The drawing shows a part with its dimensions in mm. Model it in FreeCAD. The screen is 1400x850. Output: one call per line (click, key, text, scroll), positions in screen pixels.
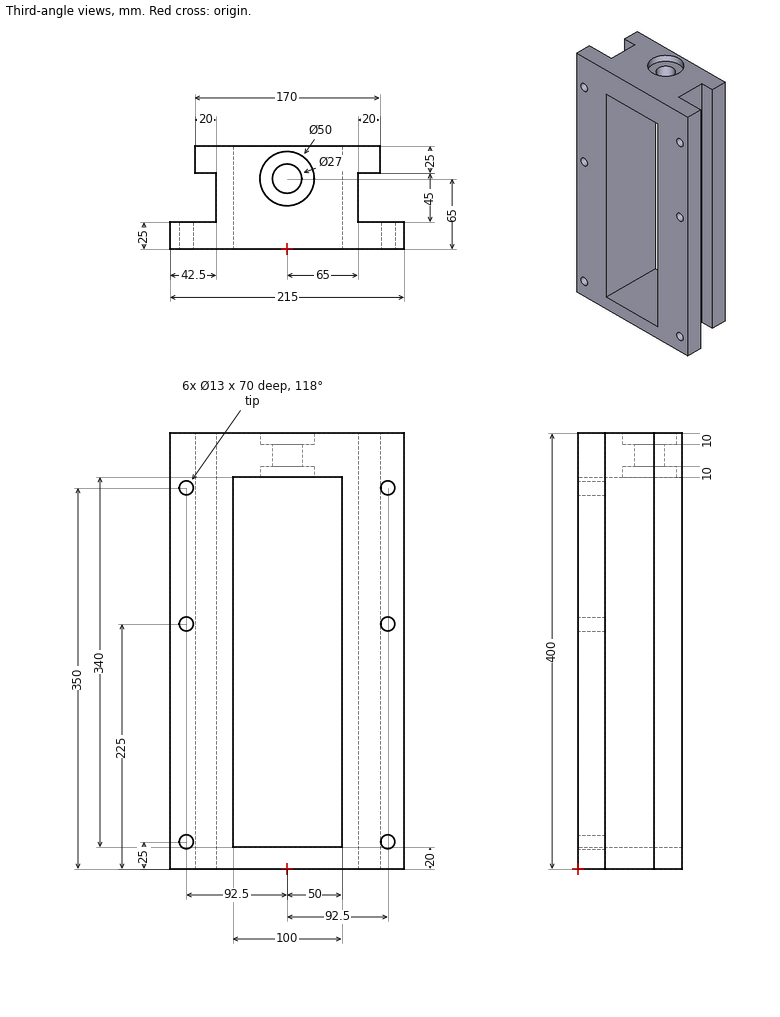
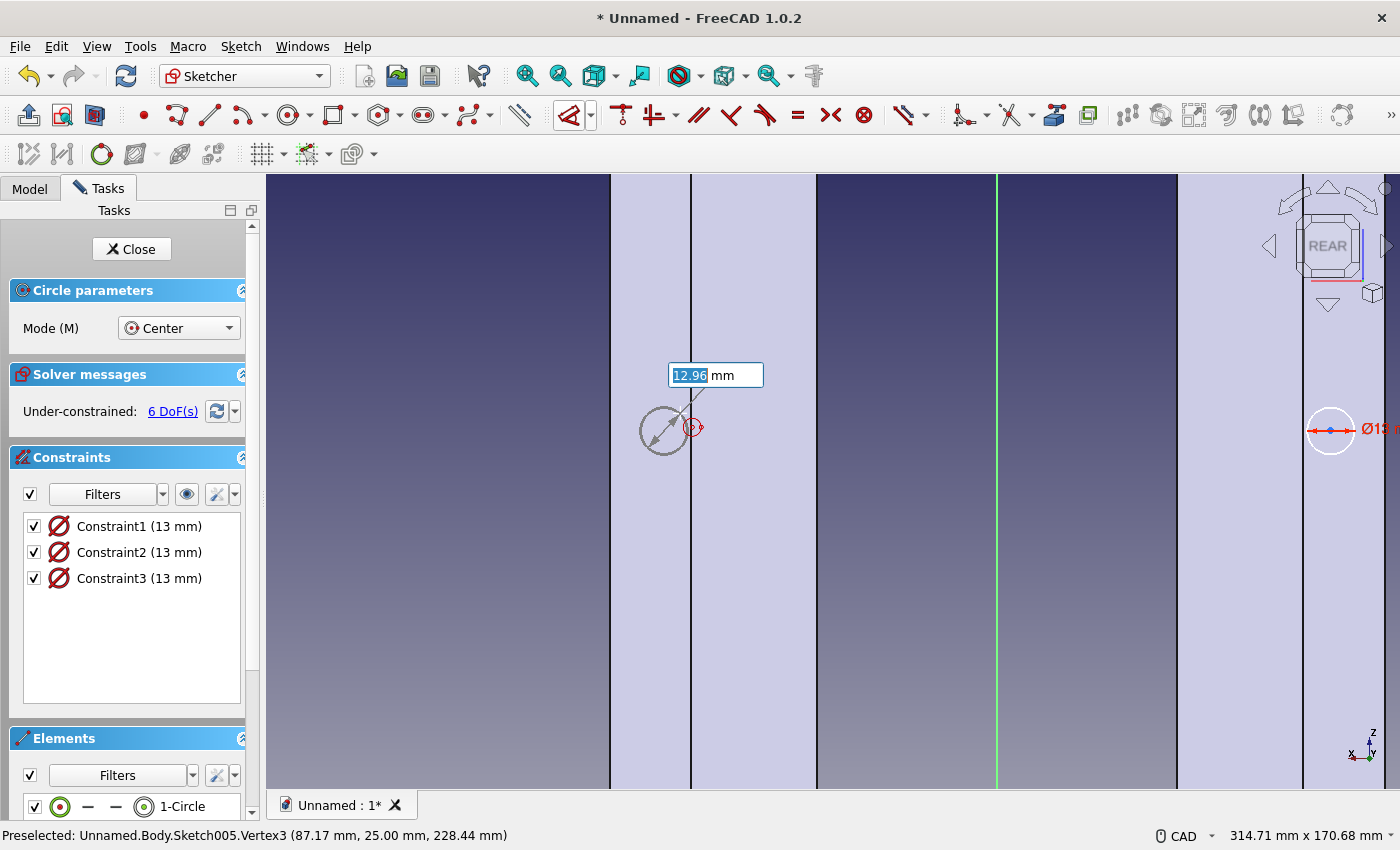
text(13)
key(Return)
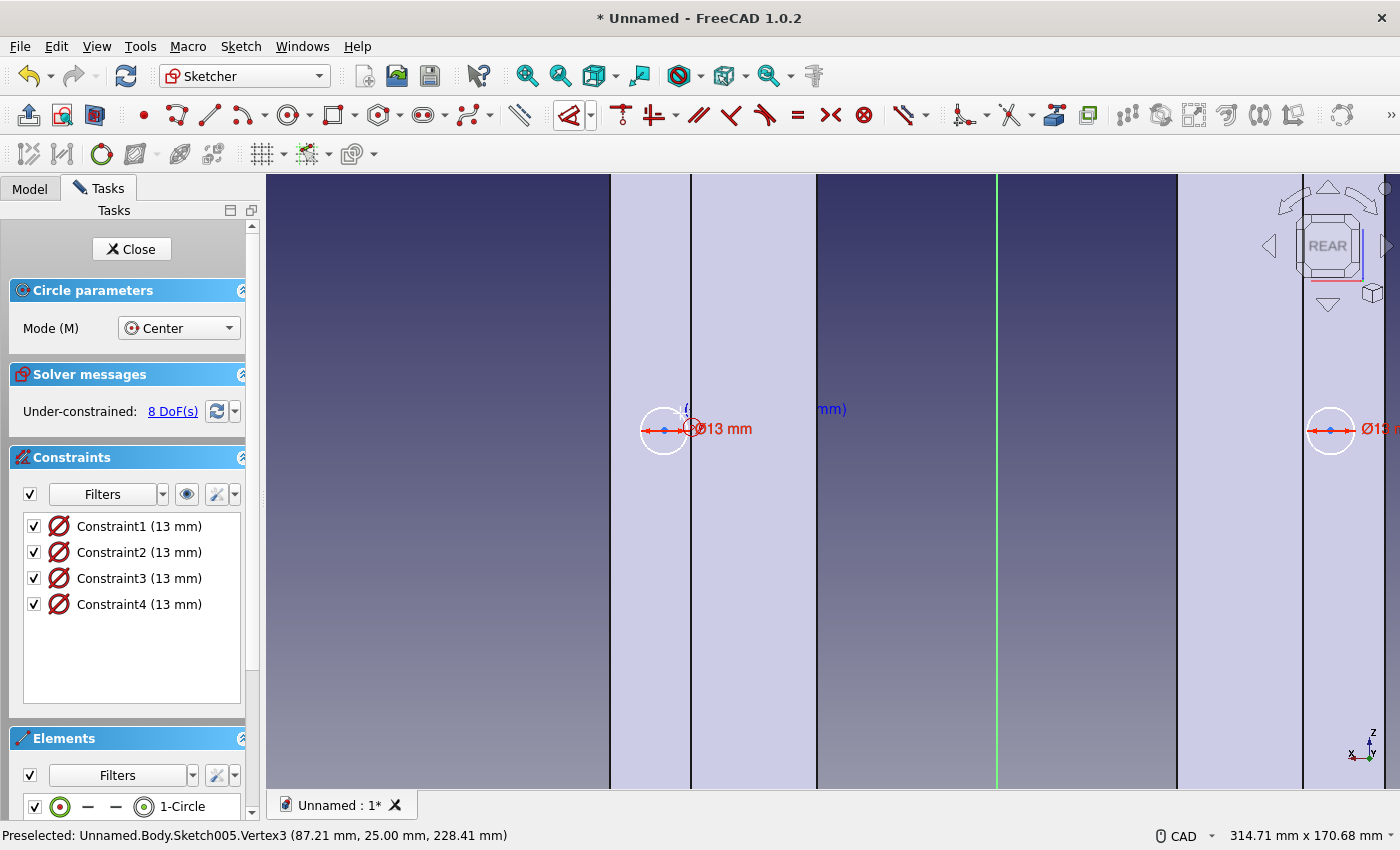
scroll(664, 431, down, 6)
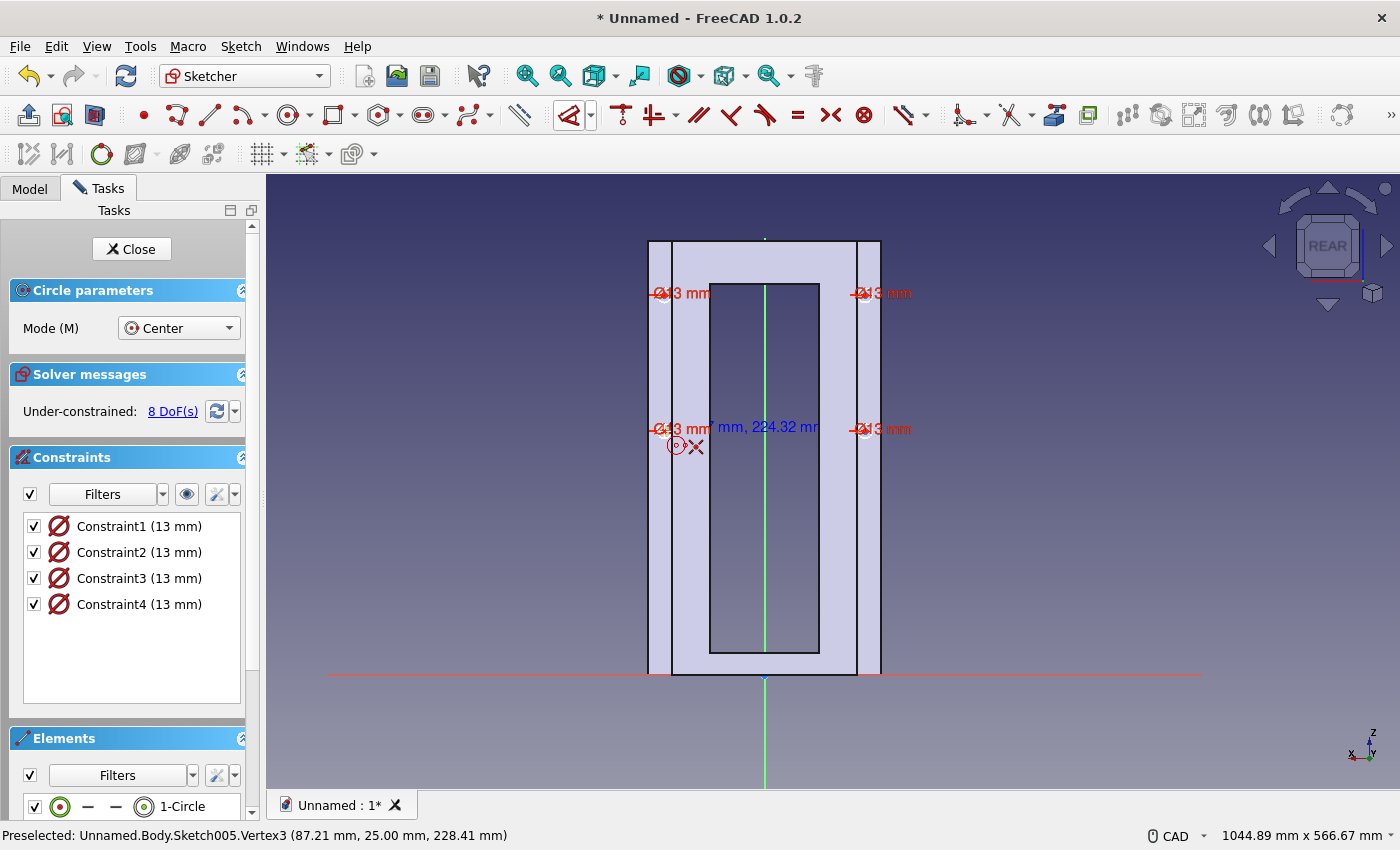
scroll(865, 648, up, 6)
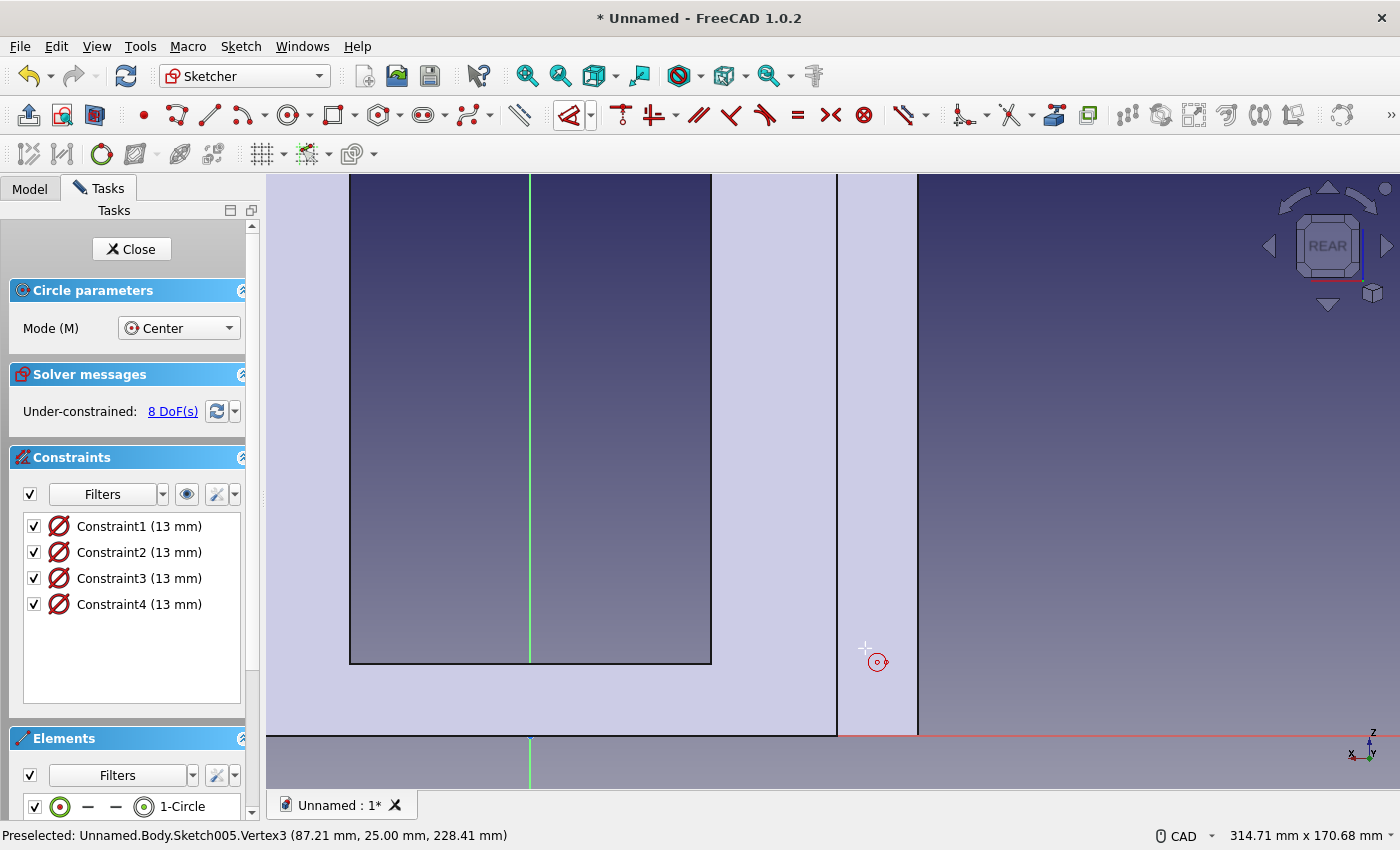
click(864, 646)
move(880, 629)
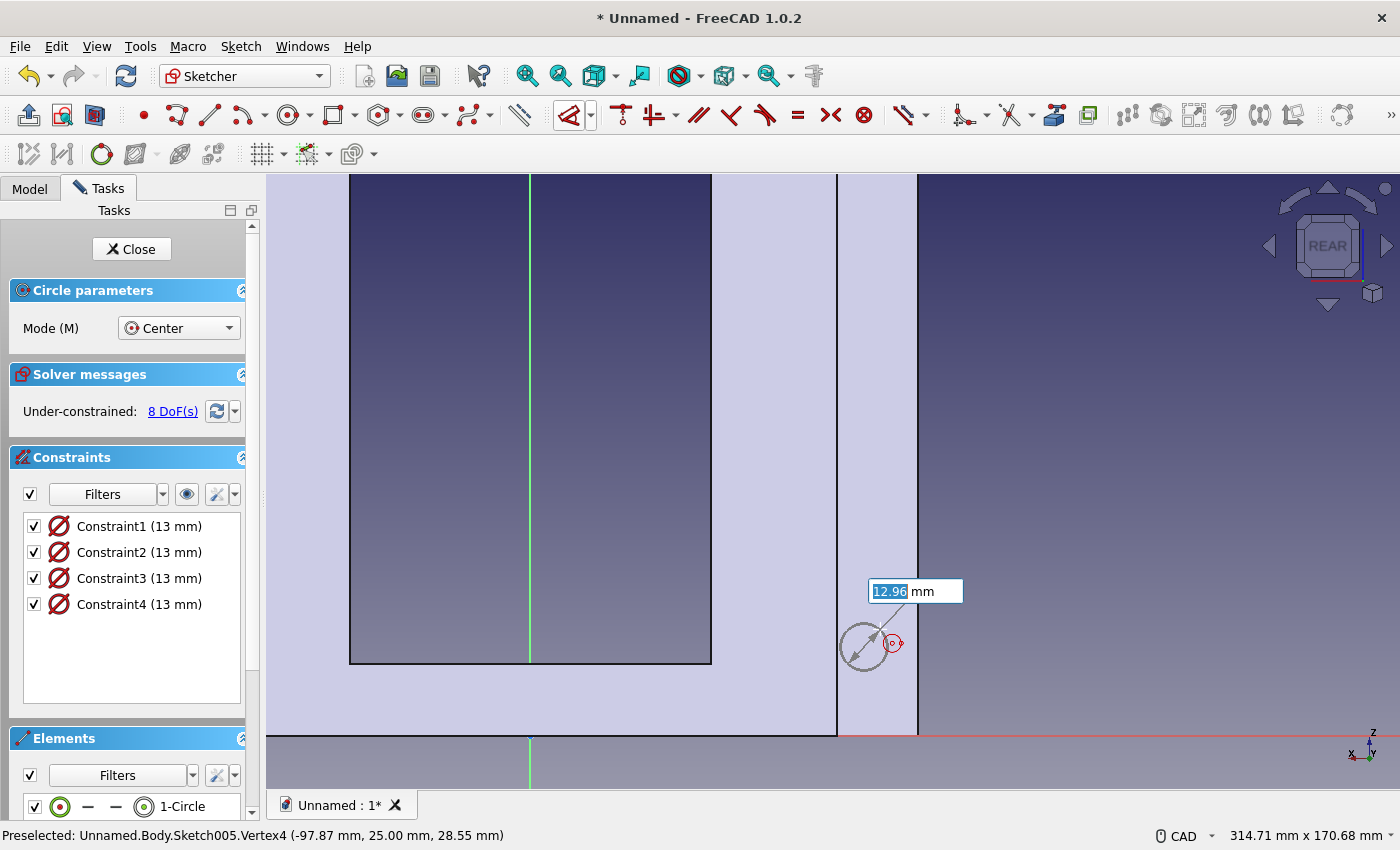
text(13)
key(Return)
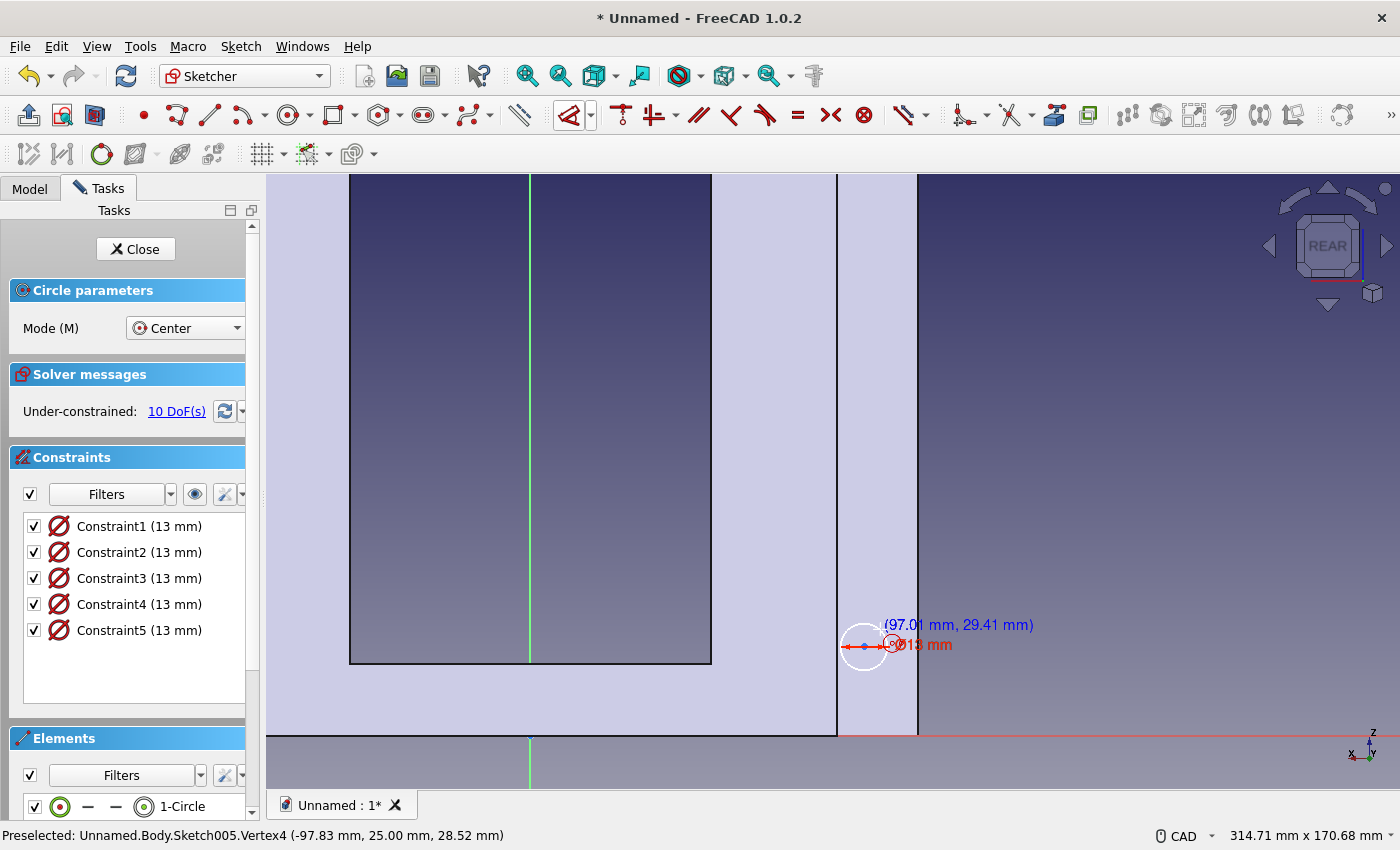
scroll(865, 649, down, 6)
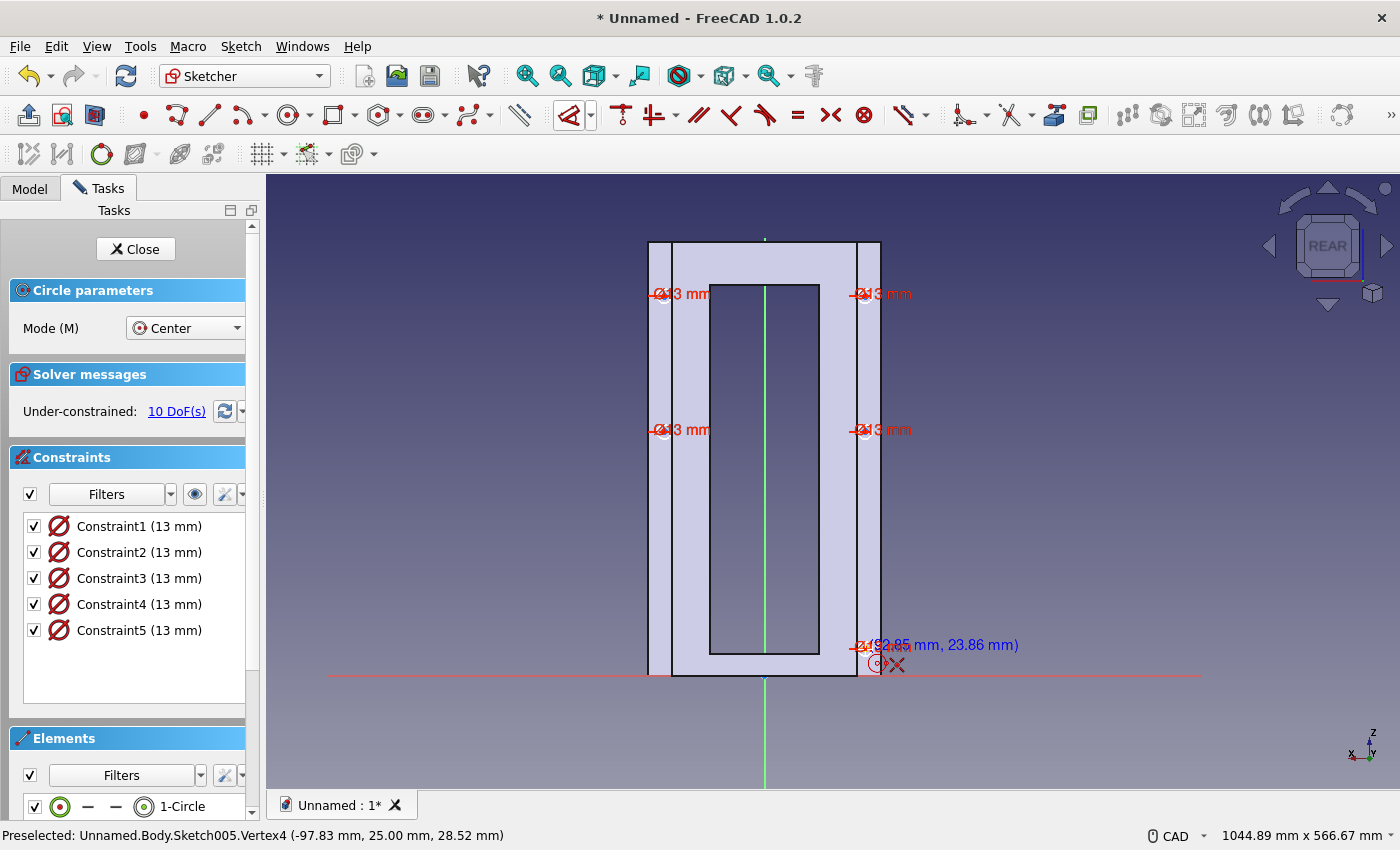
scroll(664, 649, up, 6)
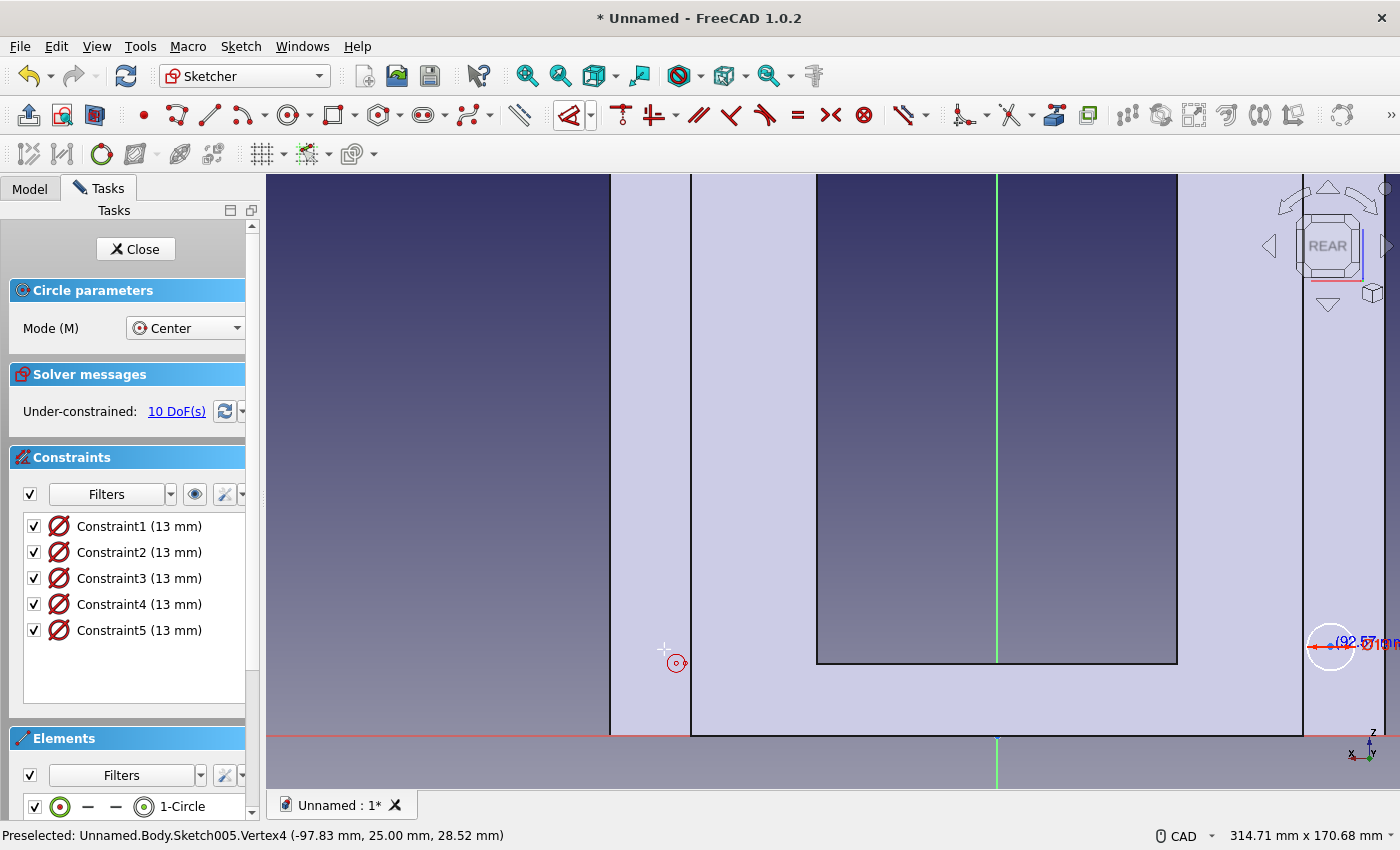
click(664, 646)
move(680, 629)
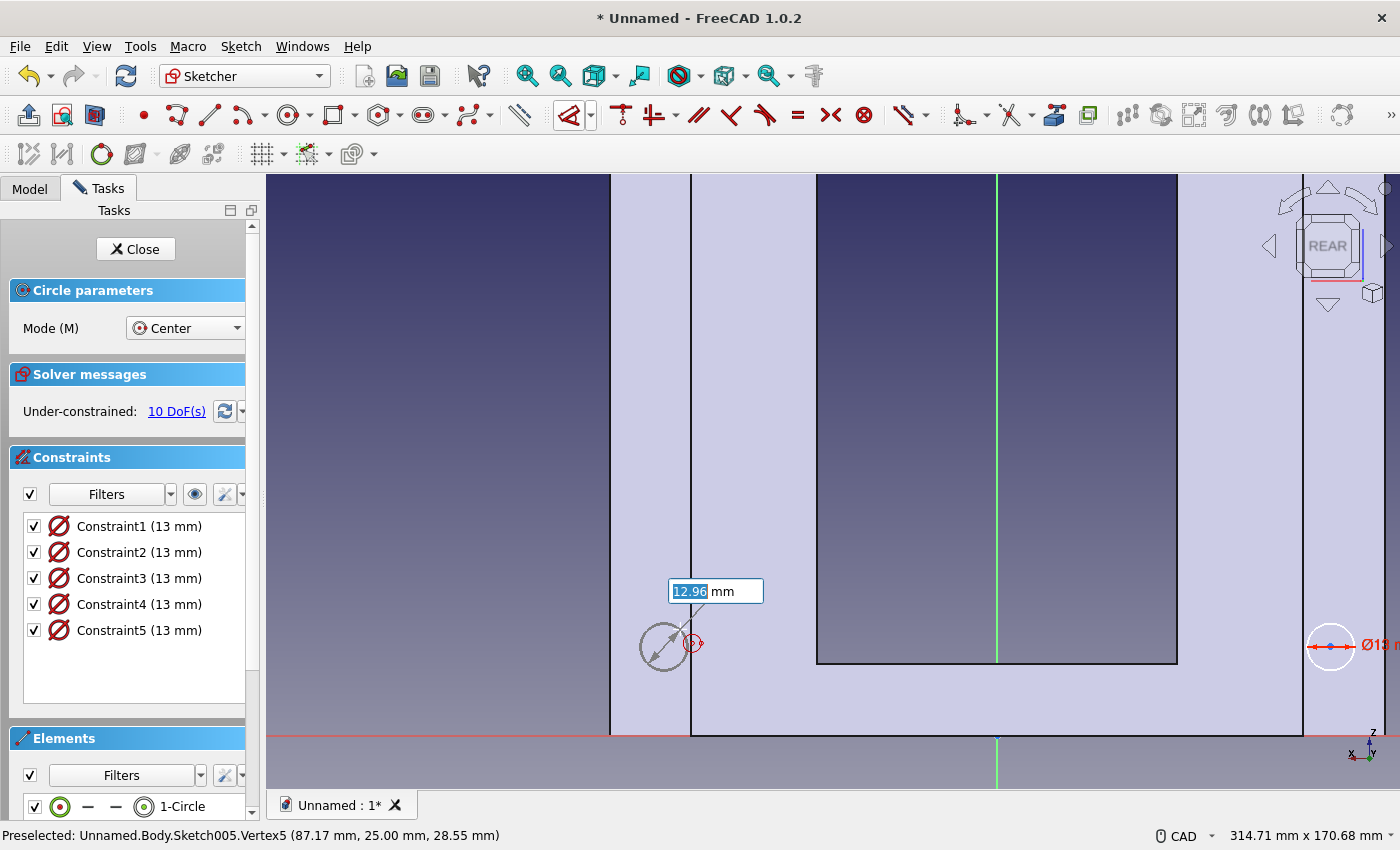
text(13)
key(Return)
key(Escape)